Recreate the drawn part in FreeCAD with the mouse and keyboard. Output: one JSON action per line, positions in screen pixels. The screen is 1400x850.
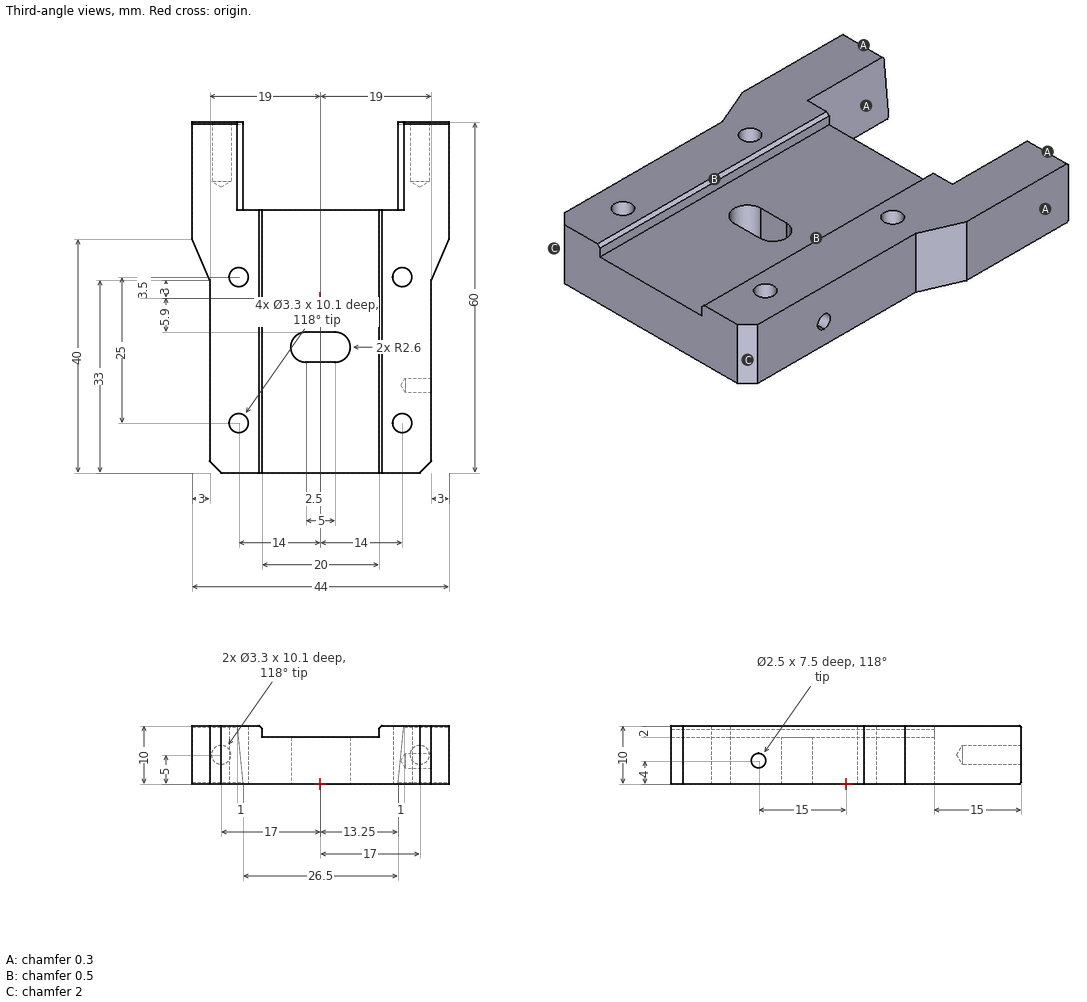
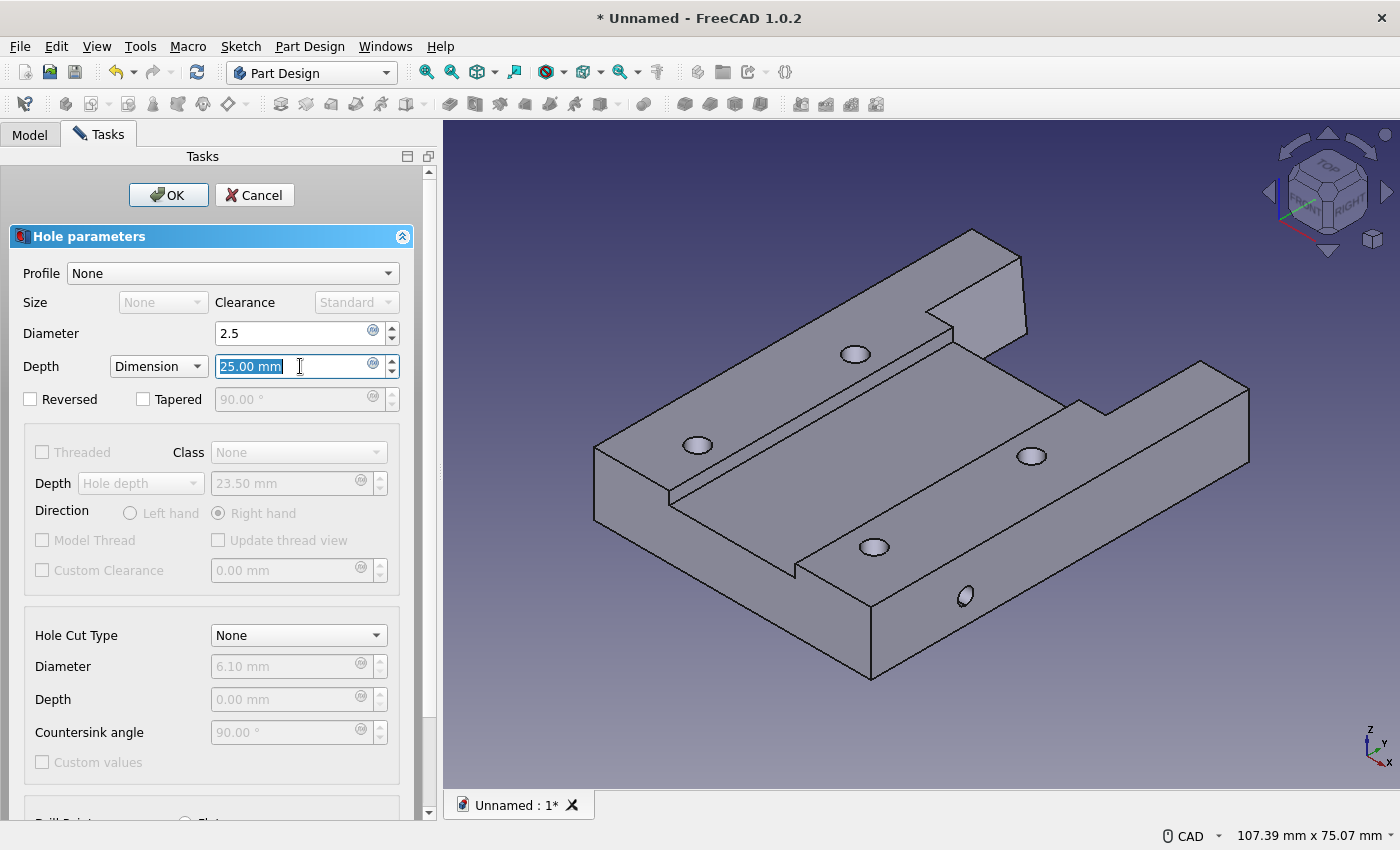
{"action": "type", "text": "7.5"}
{"action": "key", "text": "Tab"}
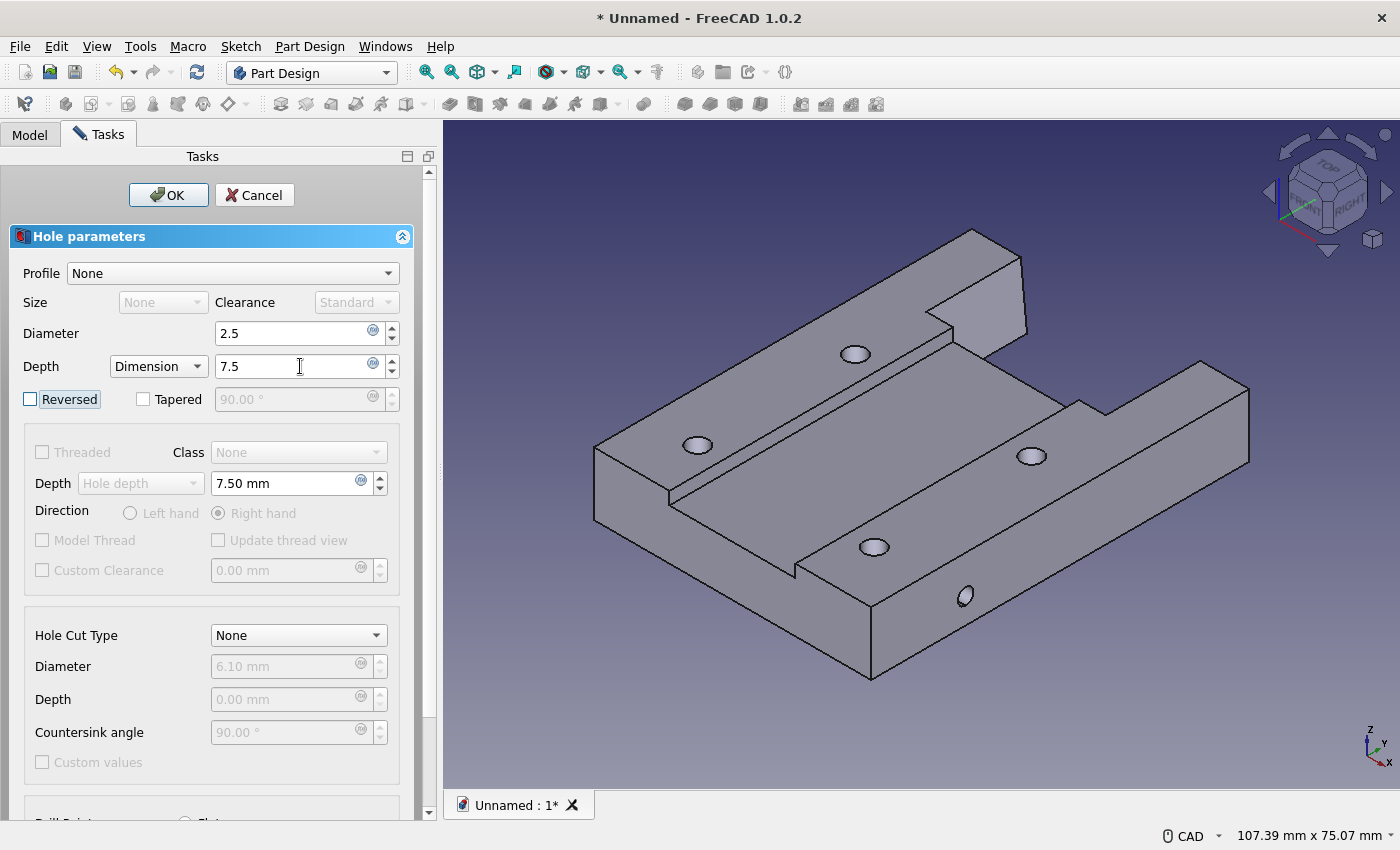
{"action": "left_click", "coordinate": [169, 195]}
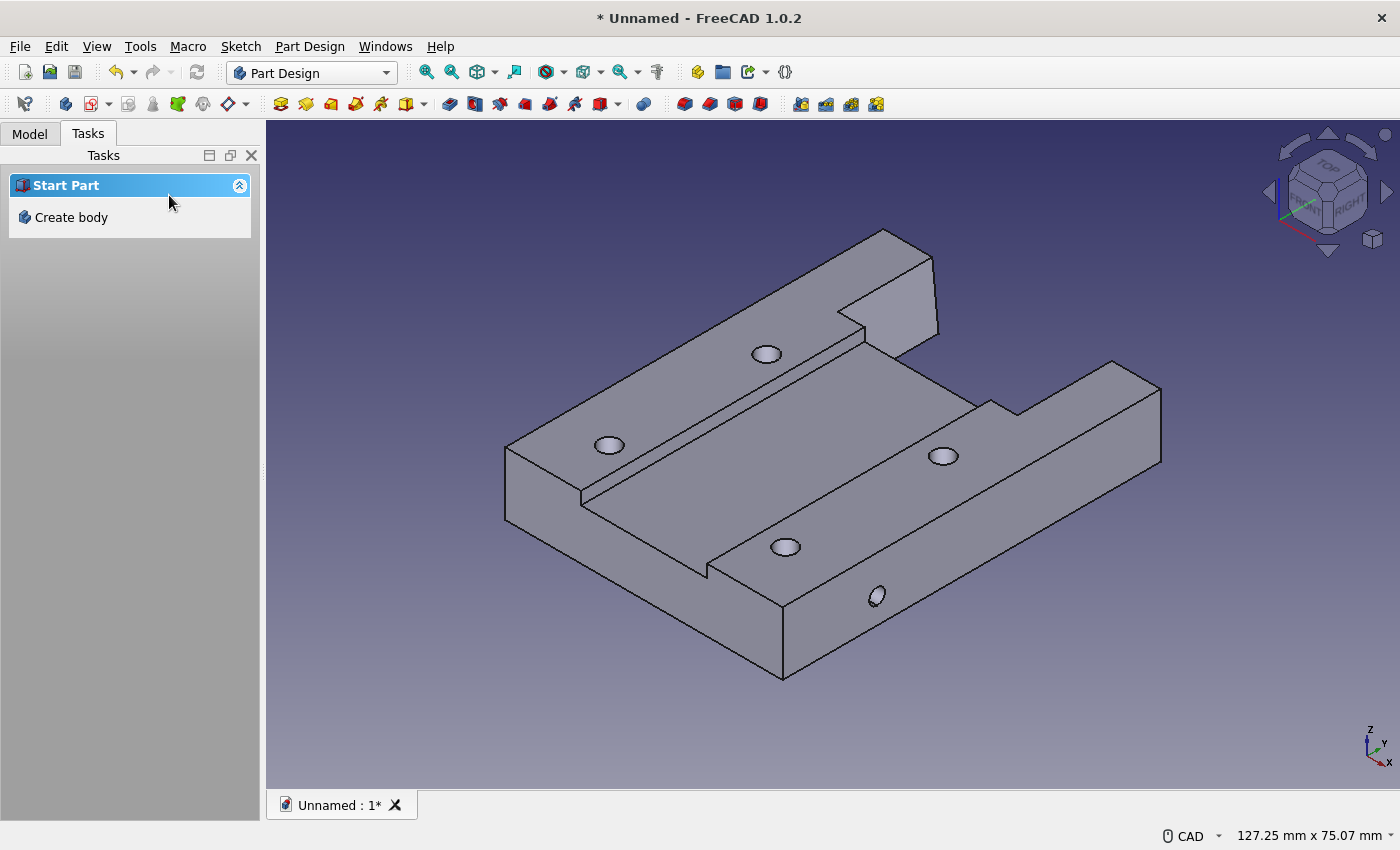
{"action": "key", "text": "2"}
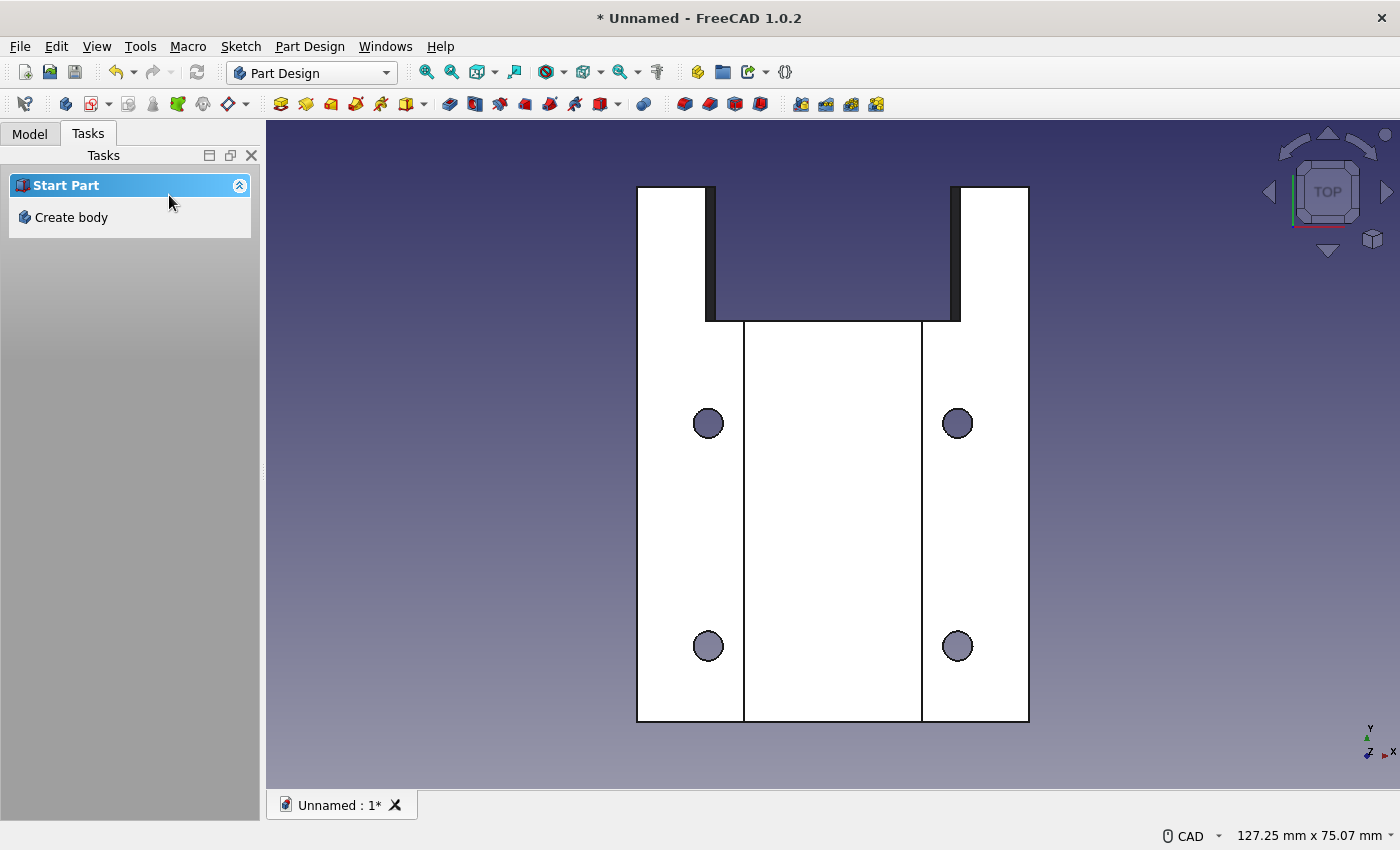
{"action": "left_click", "coordinate": [671, 186]}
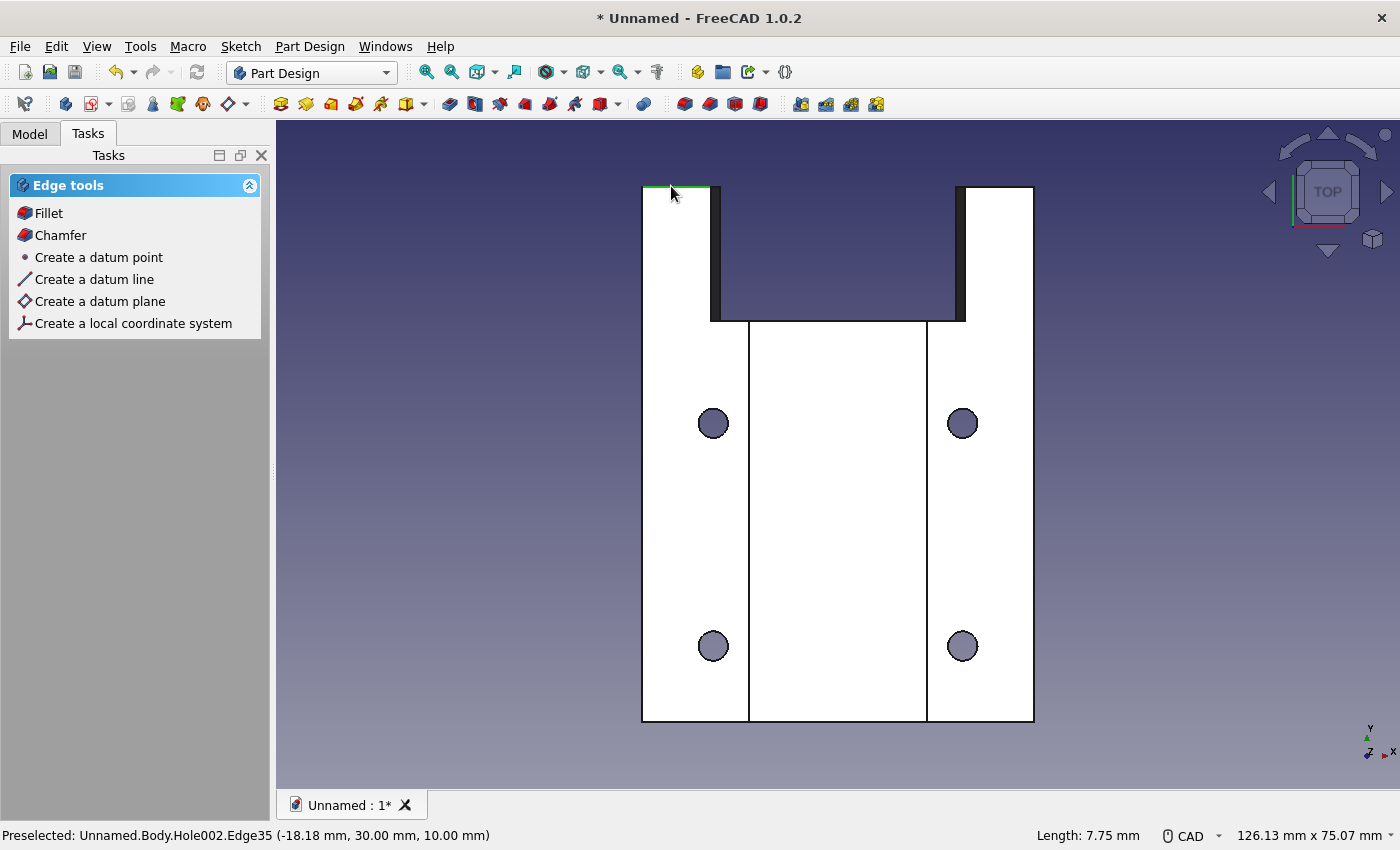
{"action": "left_click", "coordinate": [1000, 186], "text": "ctrl"}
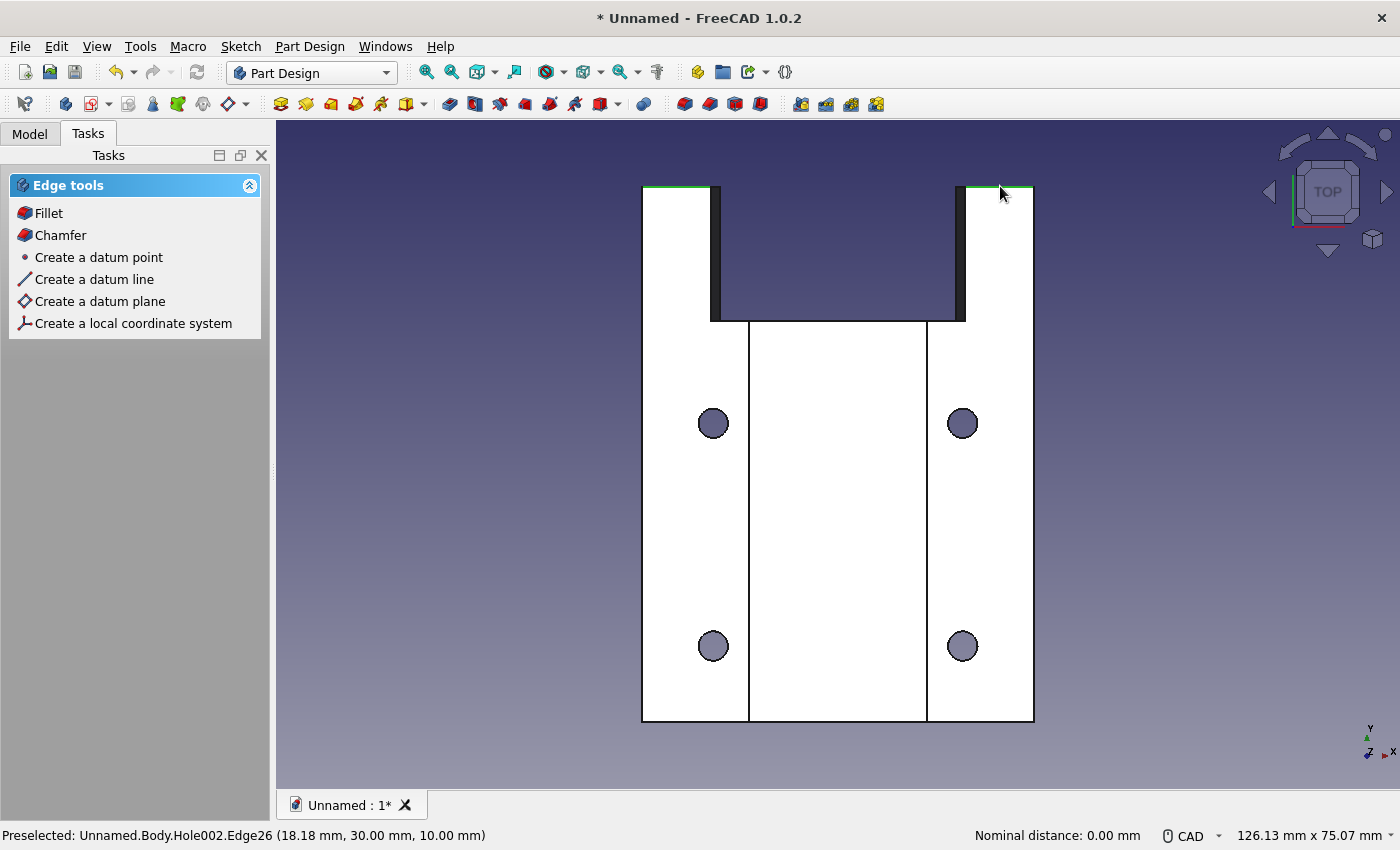
{"action": "key", "text": "0"}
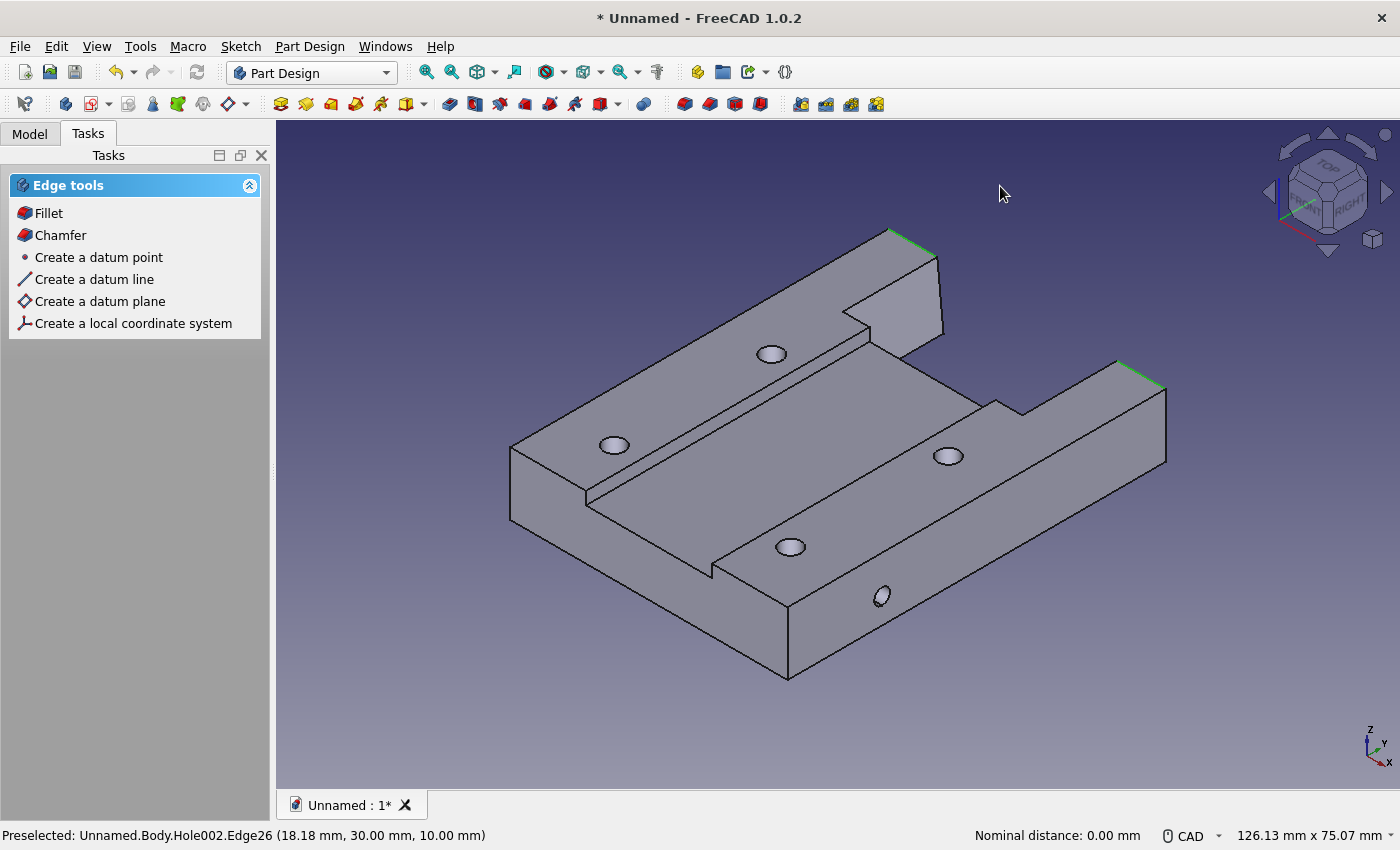
{"action": "key", "text": "1"}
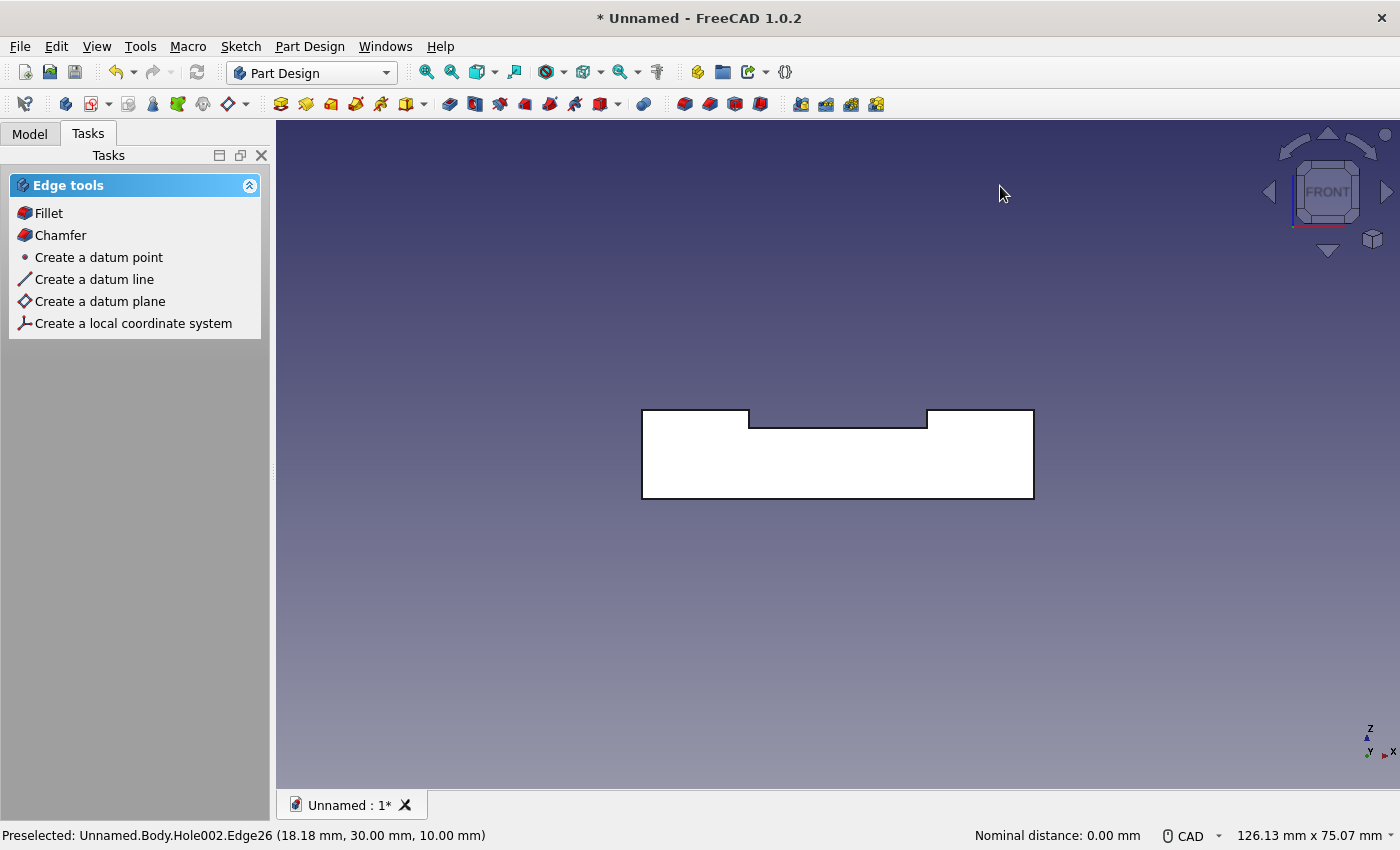
{"action": "left_click", "coordinate": [427, 72]}